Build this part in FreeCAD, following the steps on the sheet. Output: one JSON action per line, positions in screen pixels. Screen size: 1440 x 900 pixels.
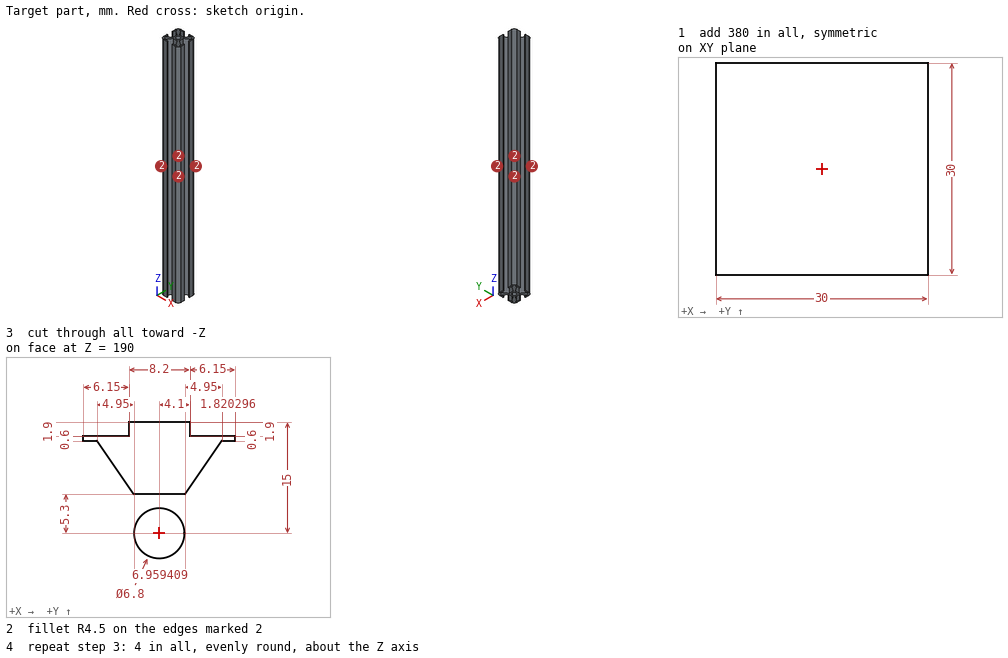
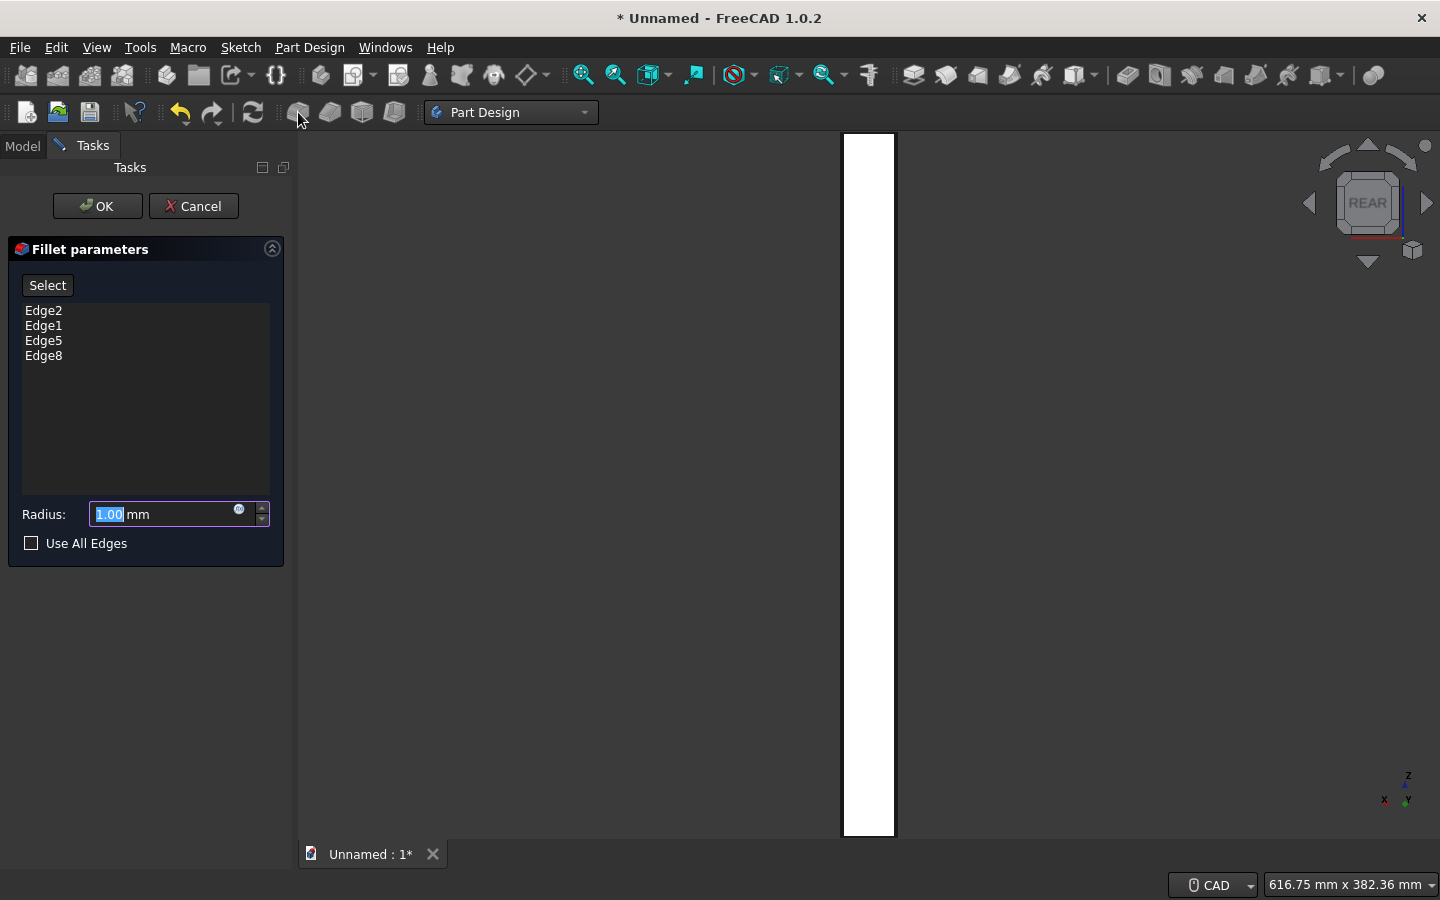
{"action": "type", "text": "4.5"}
{"action": "key", "text": "Tab"}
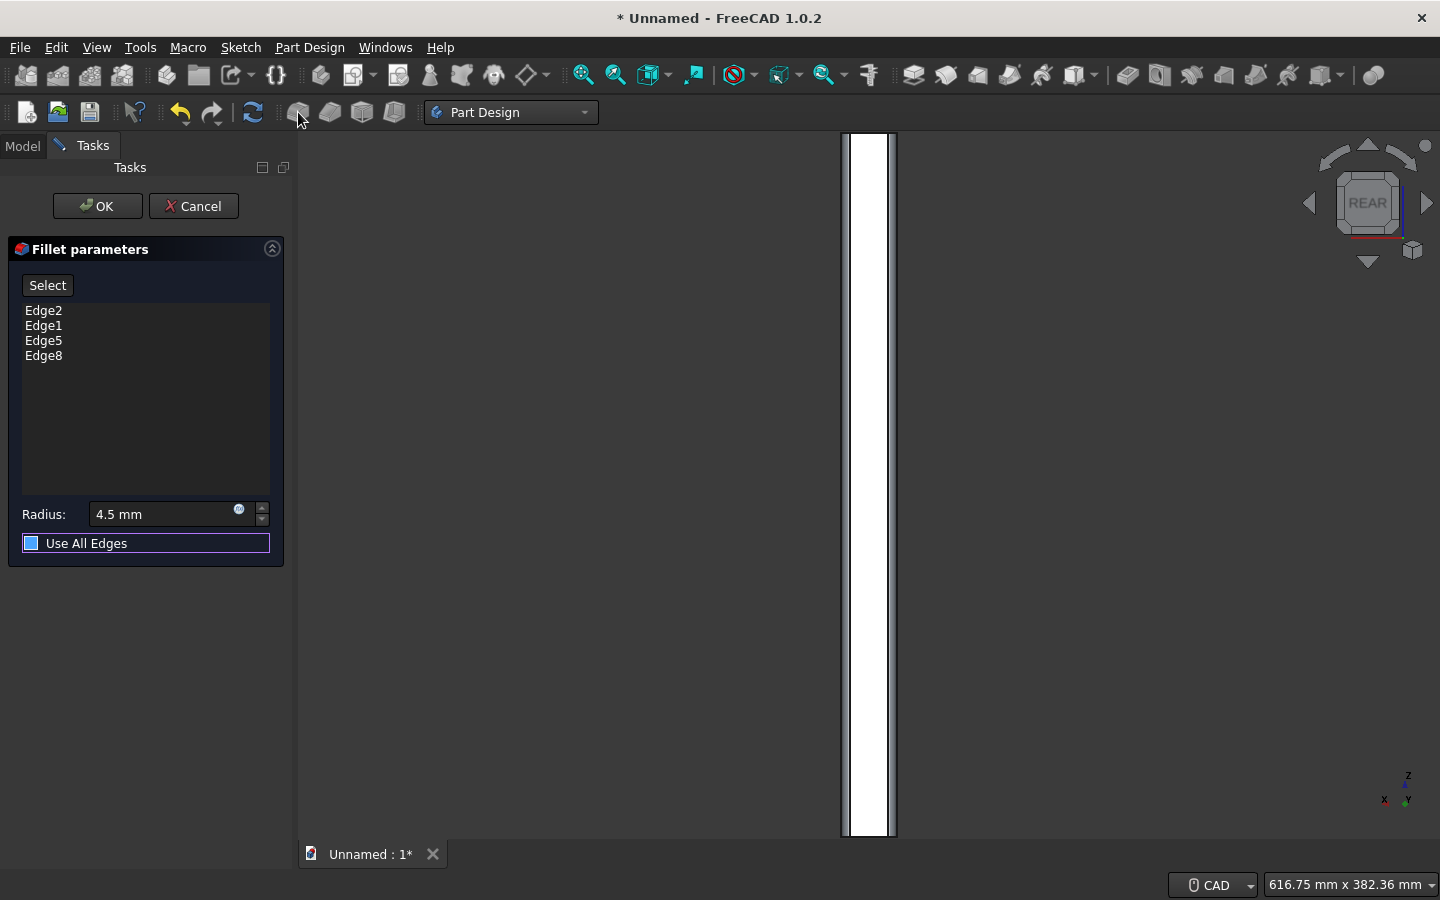
{"action": "left_click", "coordinate": [98, 206]}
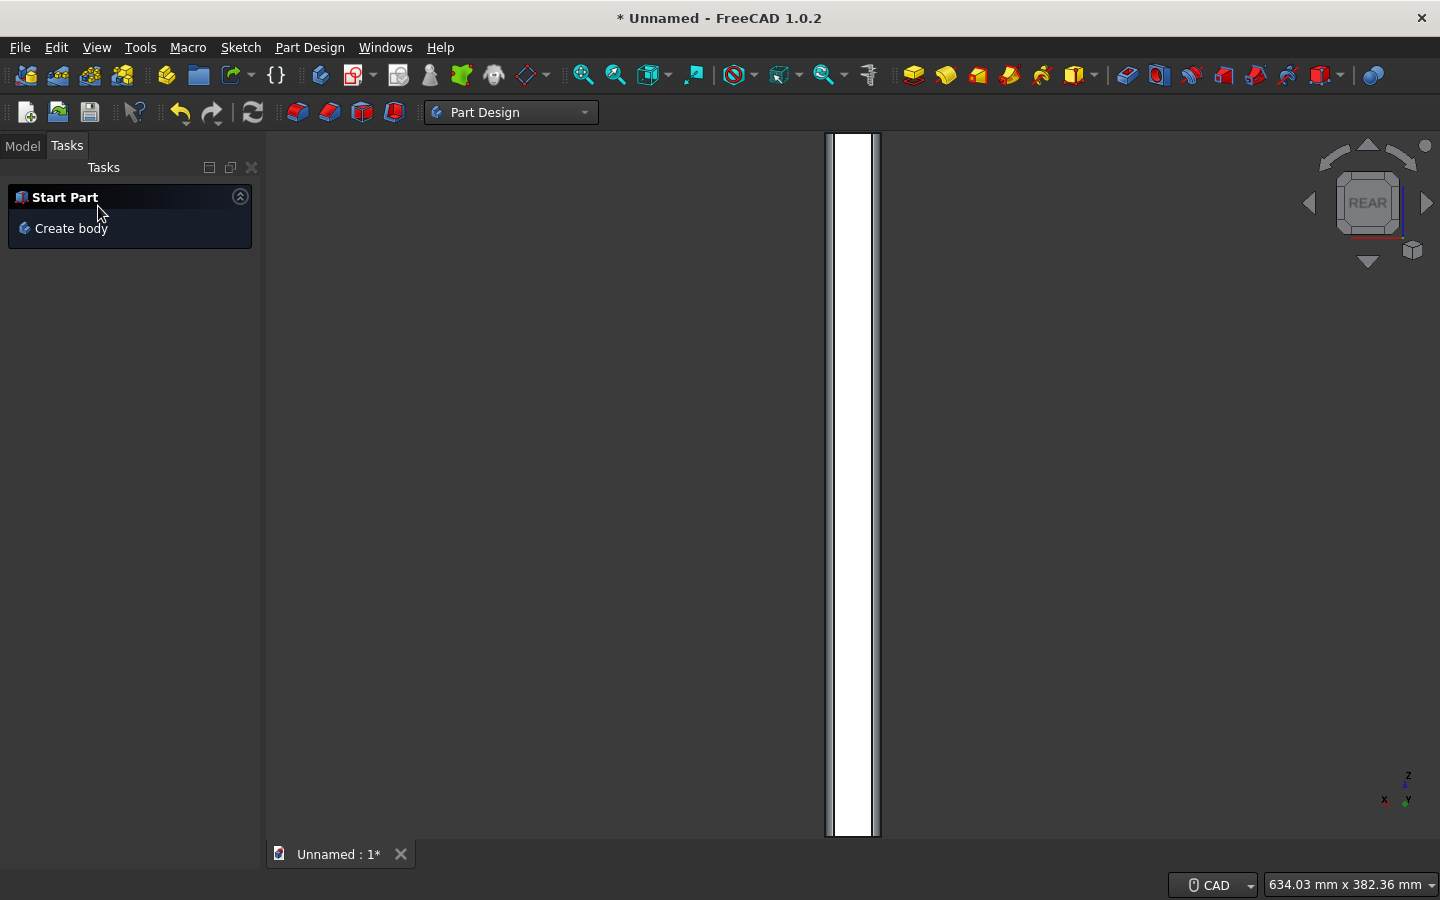
{"action": "key", "text": "0"}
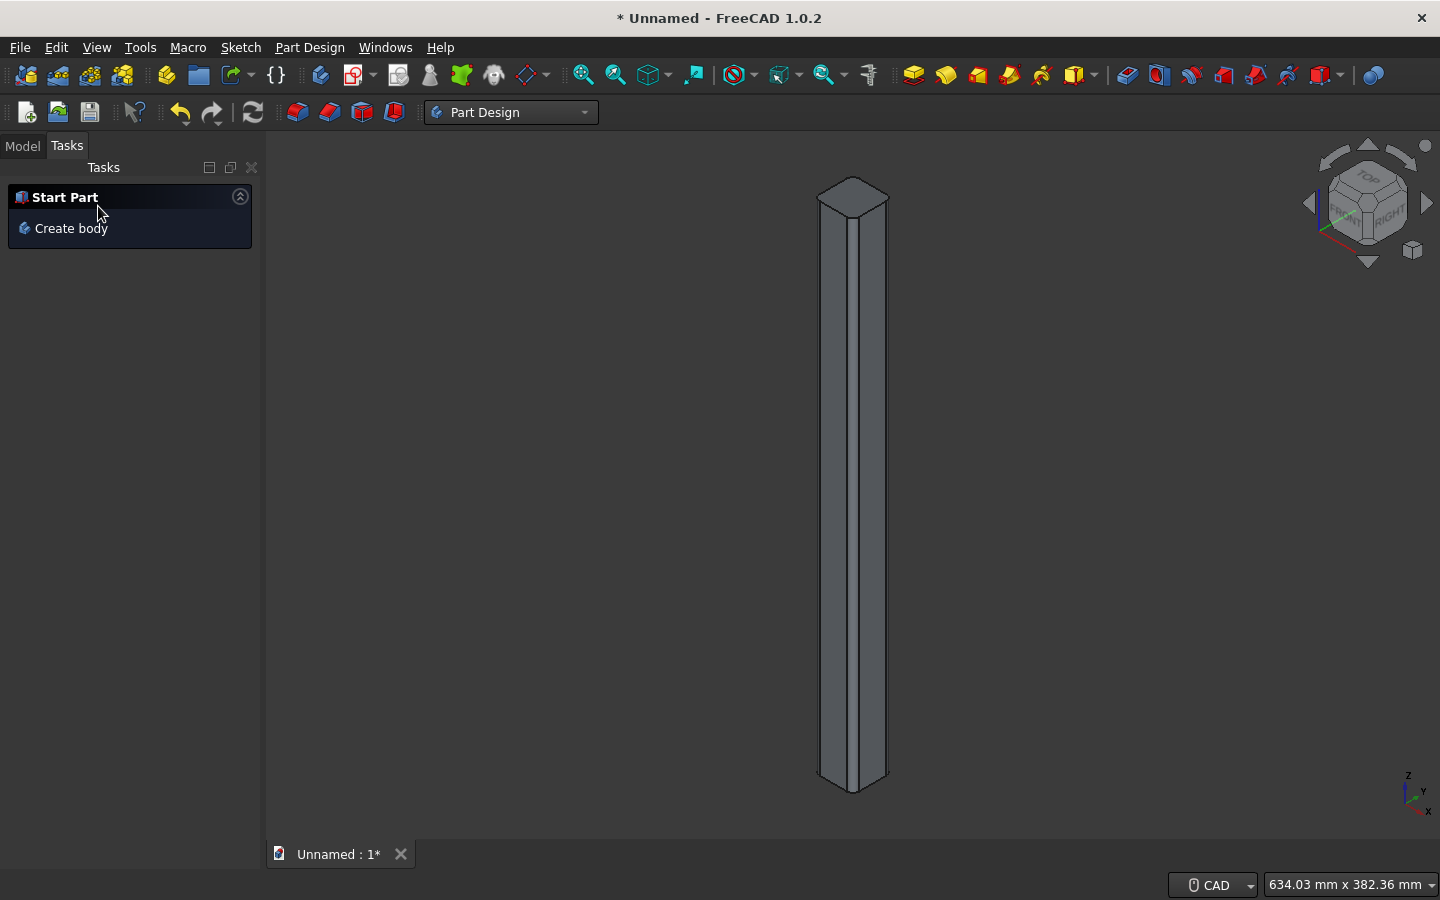
{"action": "left_click", "coordinate": [853, 197]}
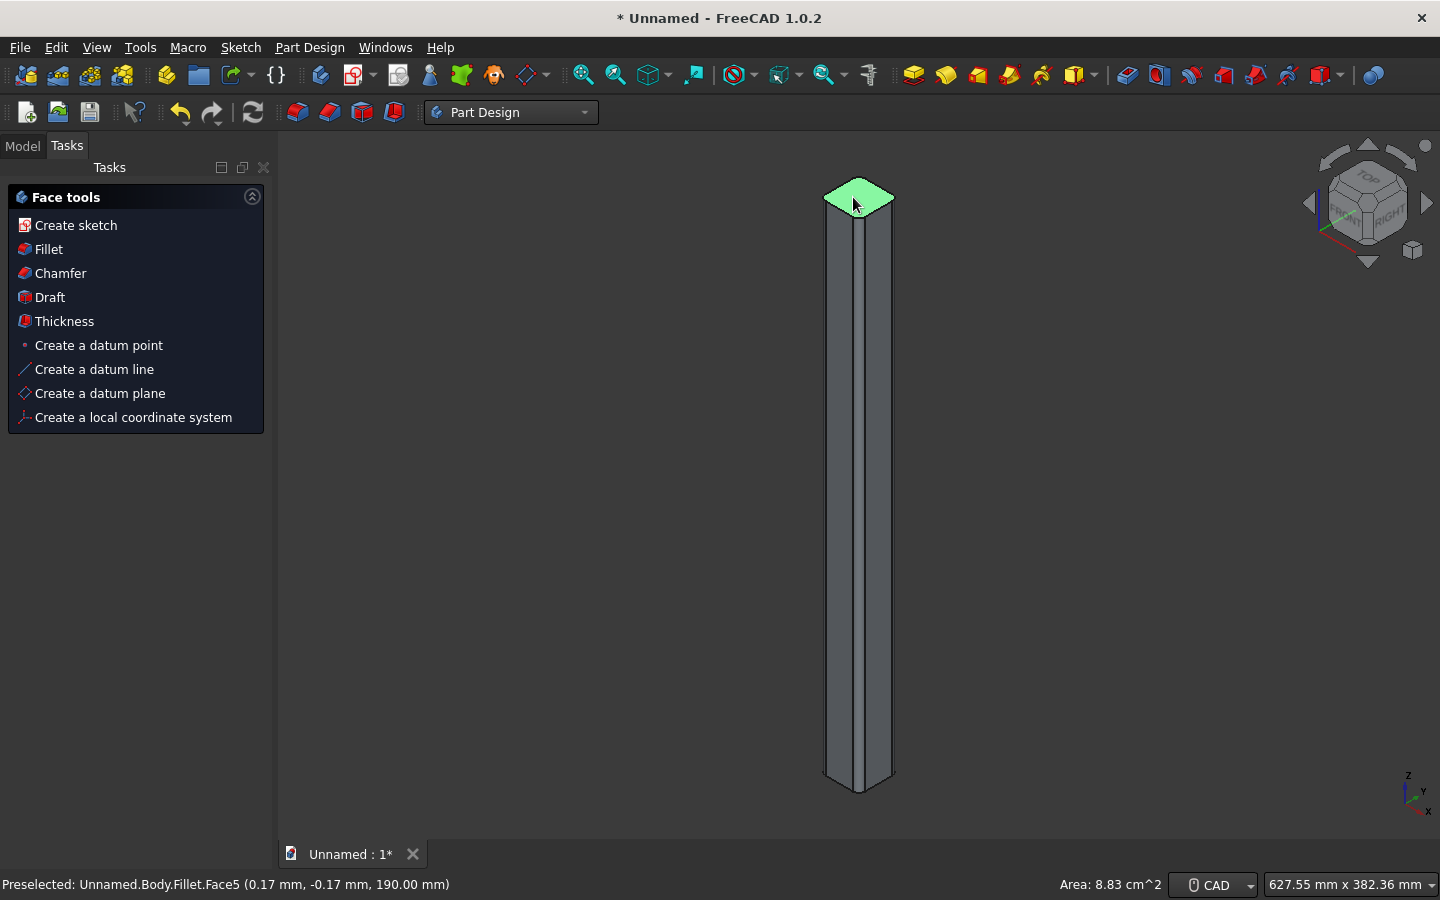
{"action": "left_click", "coordinate": [354, 76]}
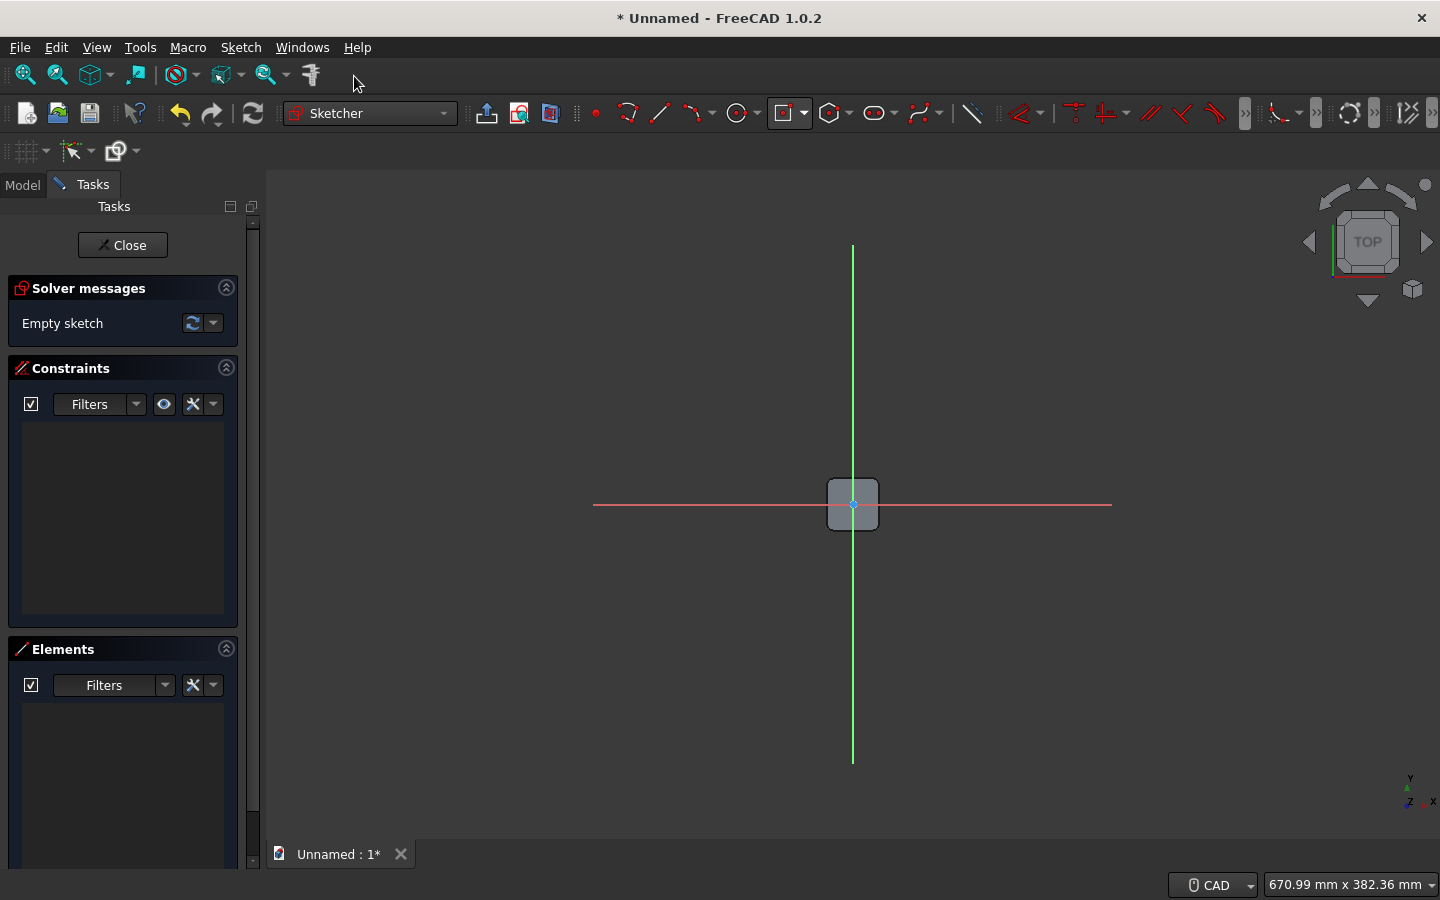
{"action": "scroll", "coordinate": [858, 494], "scroll_direction": "up", "scroll_amount": 13}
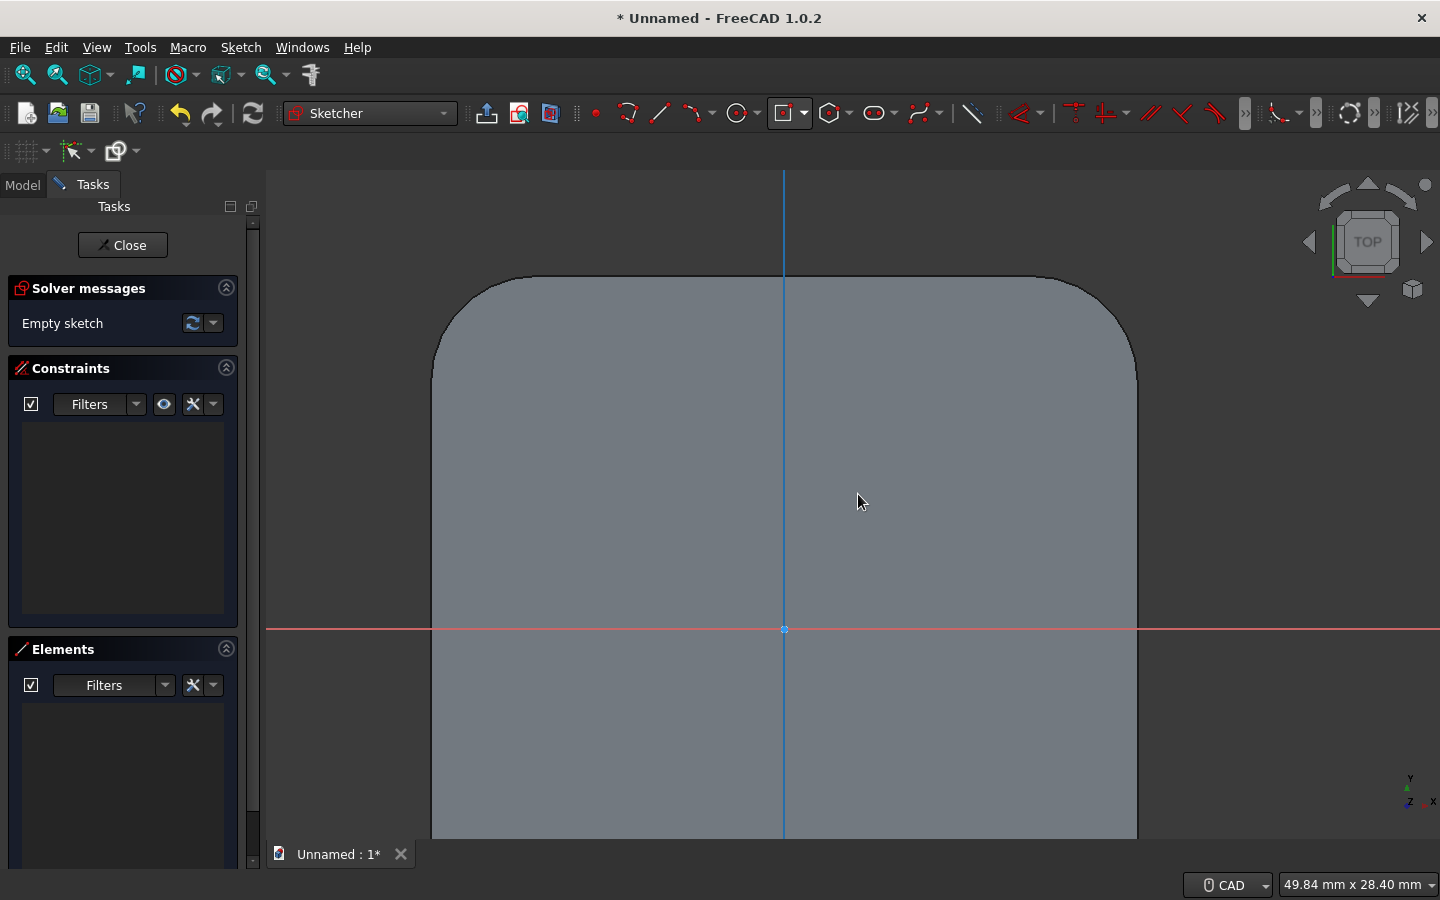
{"action": "left_click", "coordinate": [628, 114]}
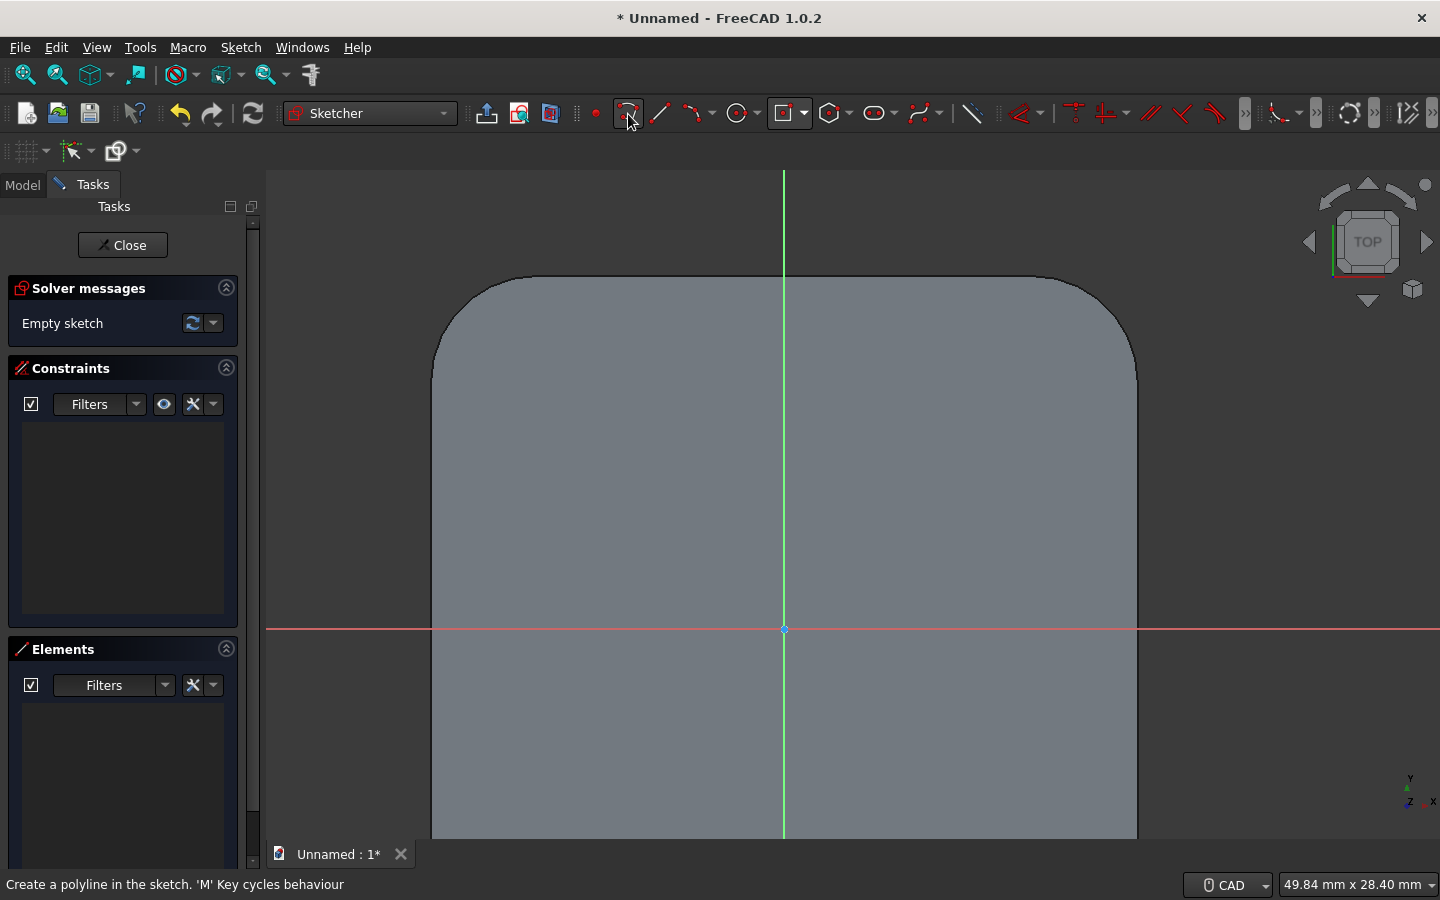
{"action": "left_click", "coordinate": [702, 504]}
{"action": "left_click", "coordinate": [866, 504]}
{"action": "left_click", "coordinate": [983, 335]}
{"action": "left_click", "coordinate": [1026, 335]}
{"action": "left_click", "coordinate": [1026, 321]}
{"action": "left_click", "coordinate": [881, 321]}
{"action": "left_click", "coordinate": [881, 276]}
{"action": "left_click", "coordinate": [688, 276]}
{"action": "left_click", "coordinate": [688, 321]}
{"action": "left_click", "coordinate": [543, 321]}
{"action": "left_click", "coordinate": [543, 335]}
{"action": "left_click", "coordinate": [586, 335]}
{"action": "left_click", "coordinate": [702, 505]}